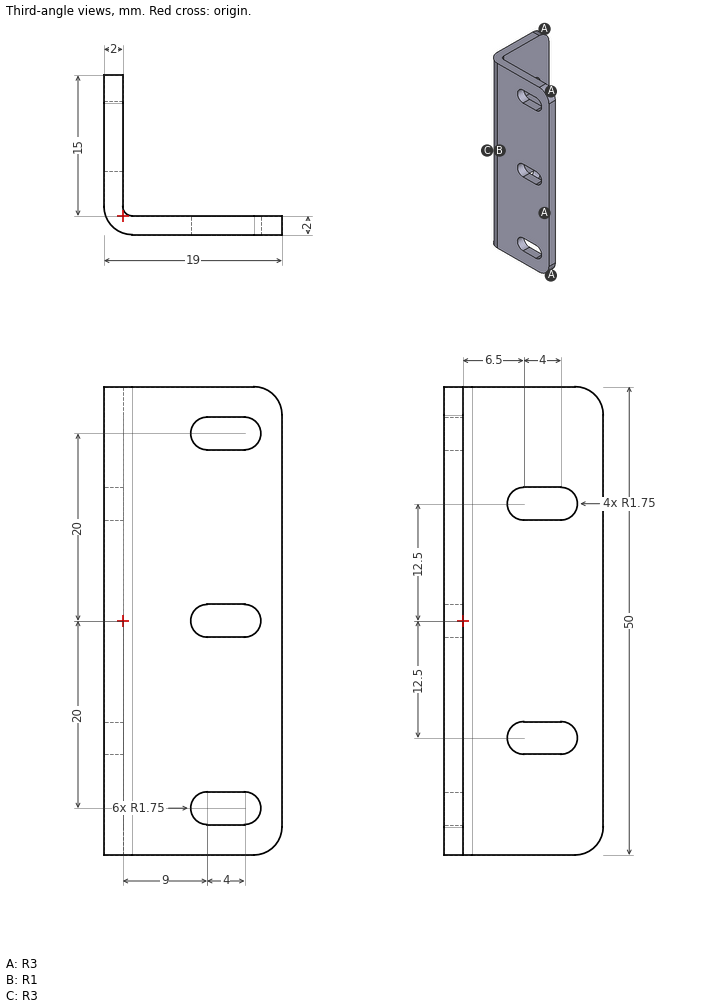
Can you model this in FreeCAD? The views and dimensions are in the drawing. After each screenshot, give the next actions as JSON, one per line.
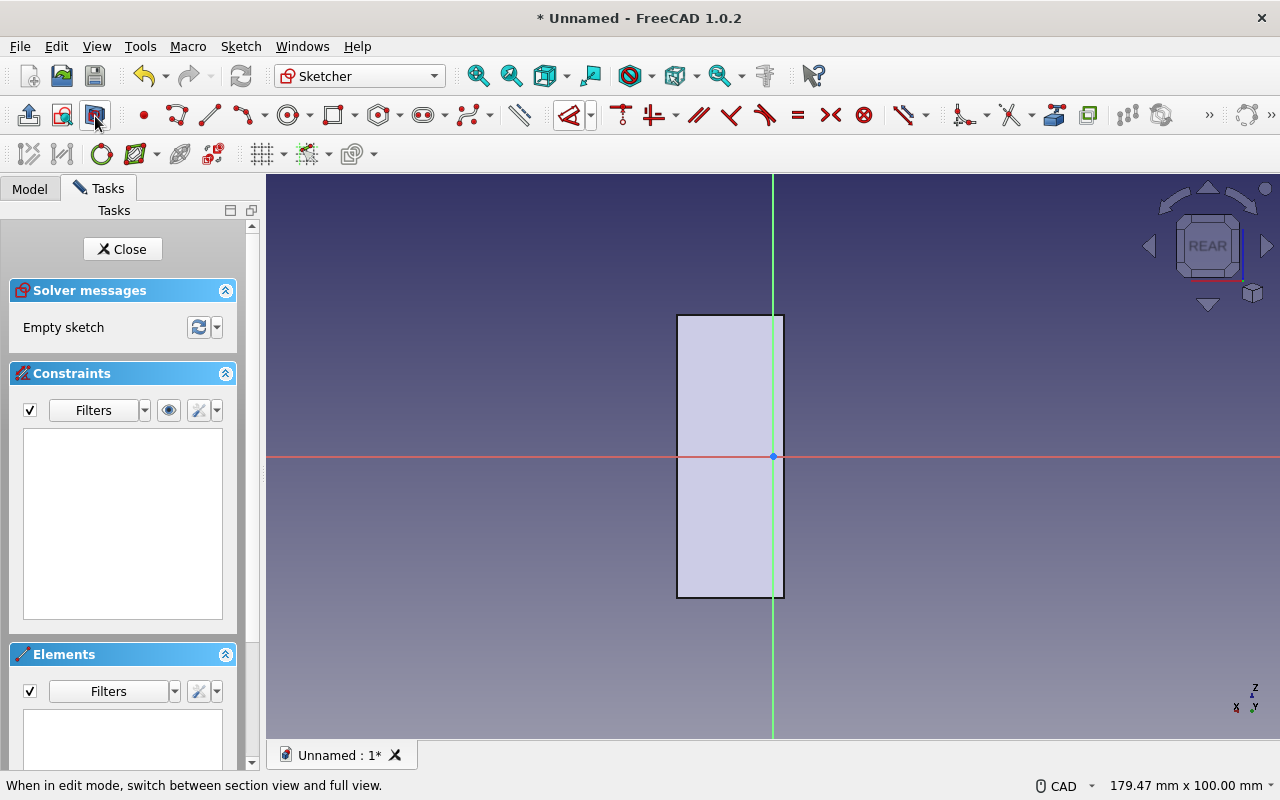
{"action": "scroll", "coordinate": [786, 456], "scroll_direction": "up", "scroll_amount": 2}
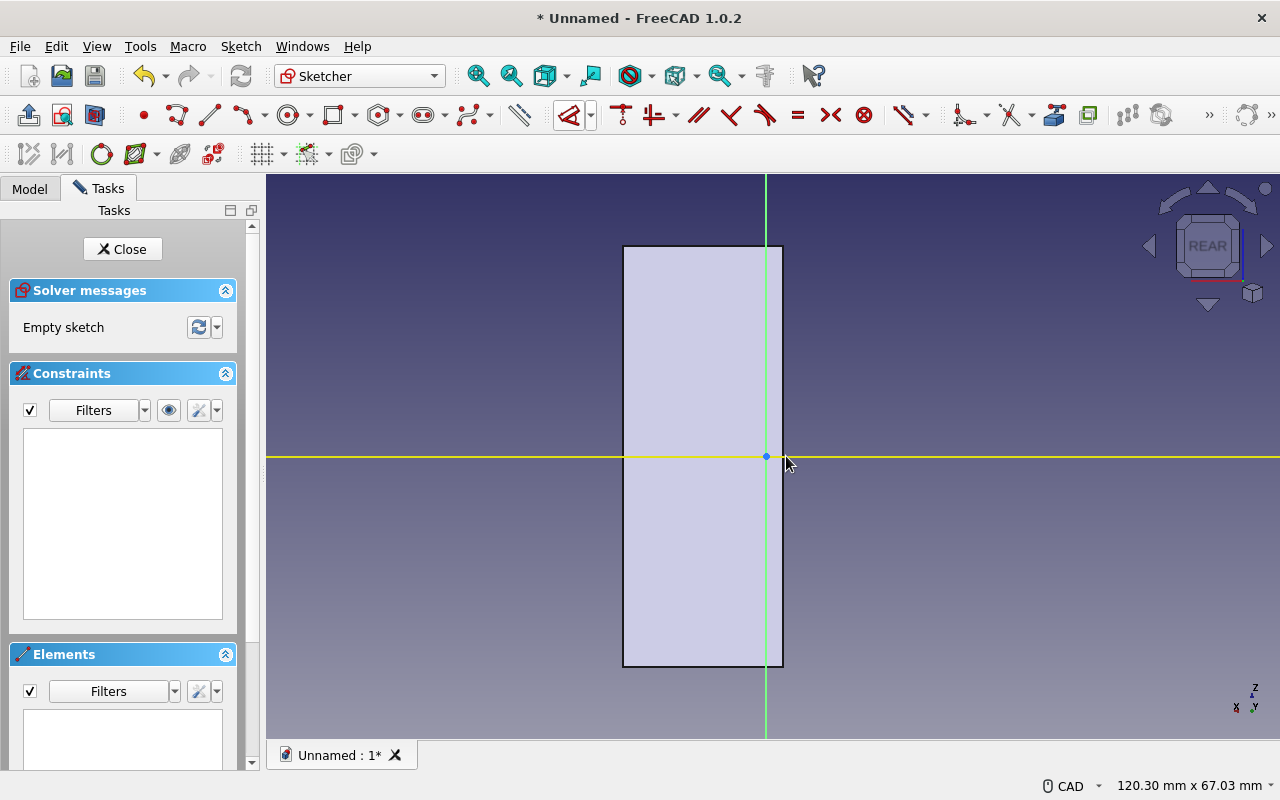
{"action": "key", "text": "g s"}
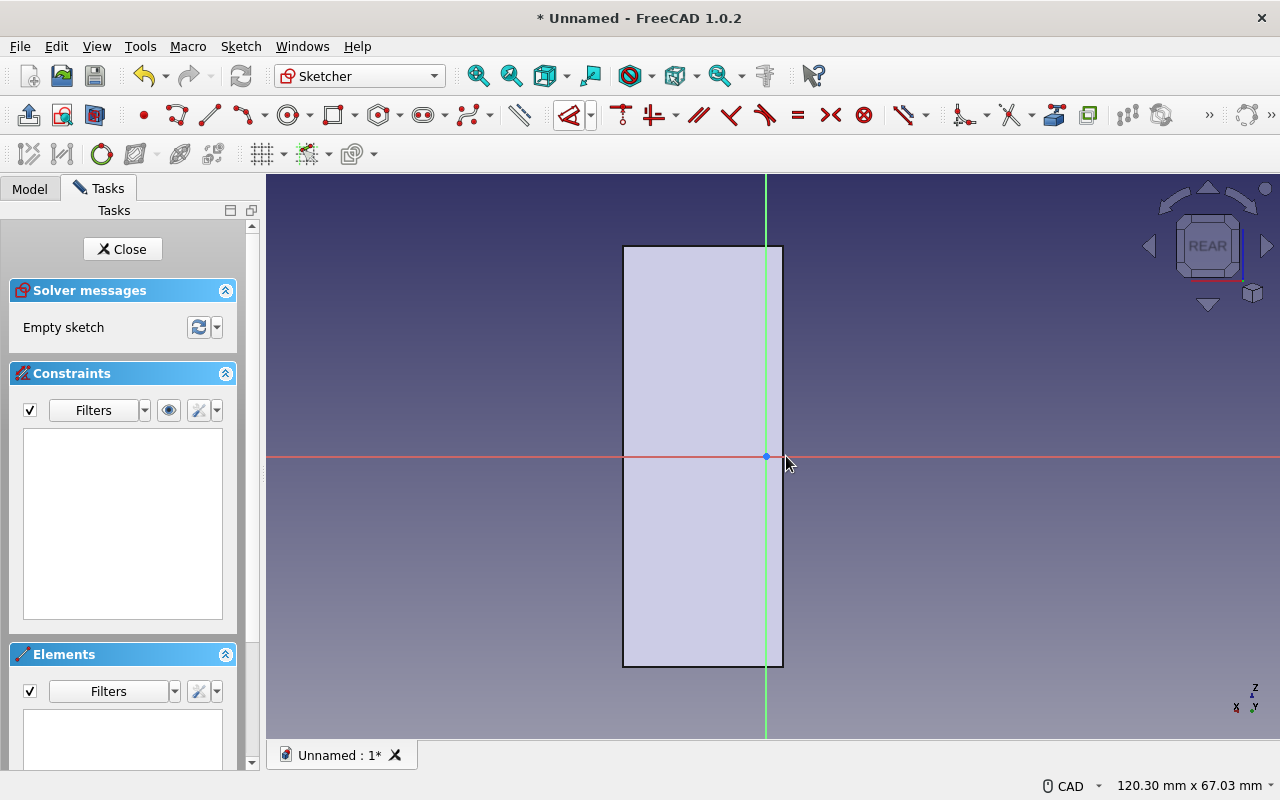
{"action": "scroll", "coordinate": [657, 625], "scroll_direction": "up", "scroll_amount": 3}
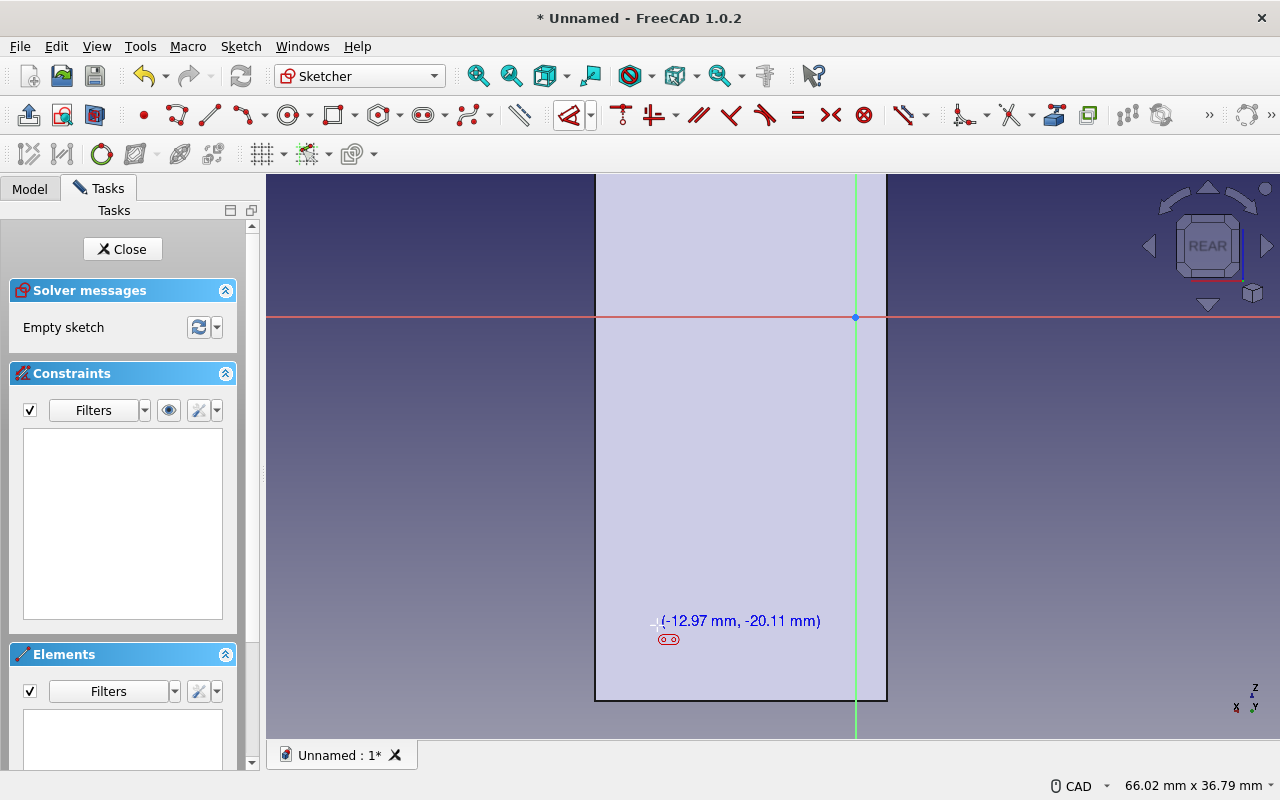
{"action": "left_click", "coordinate": [656, 624]}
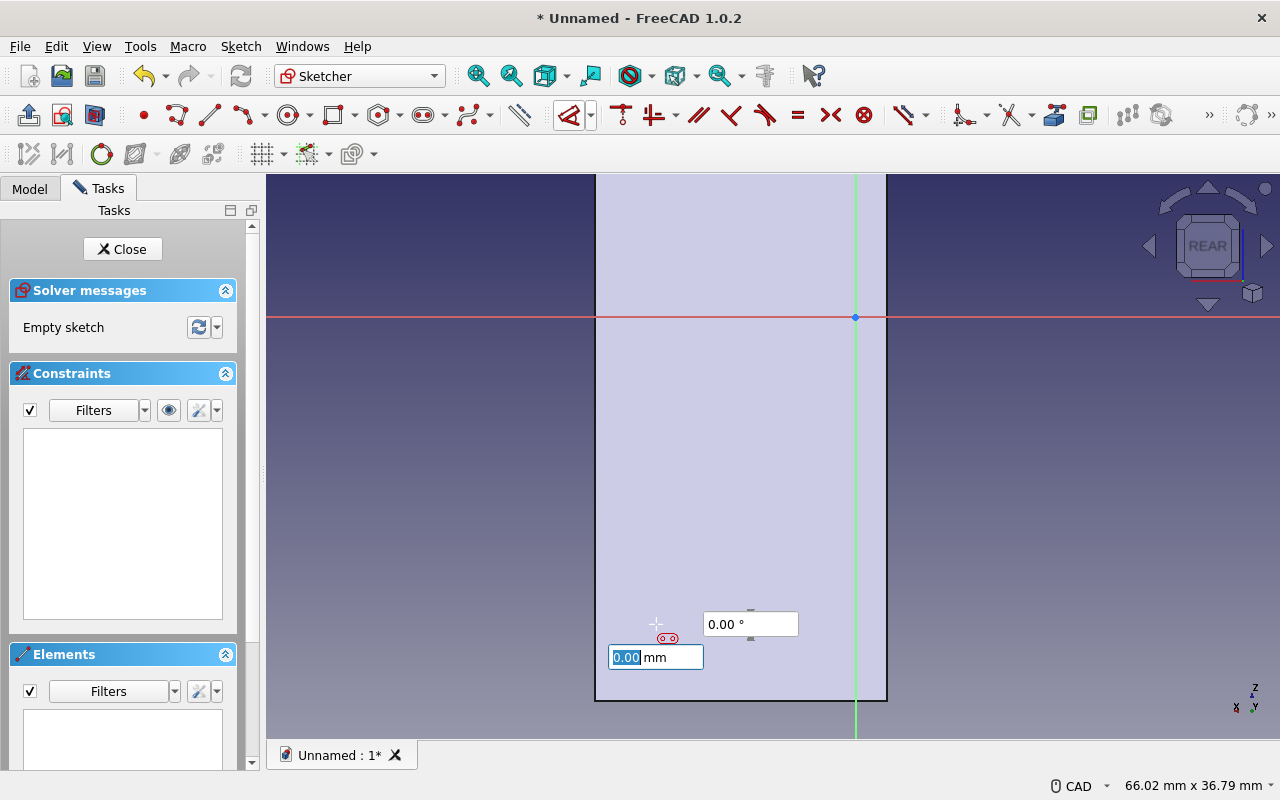
{"action": "left_click", "coordinate": [718, 624]}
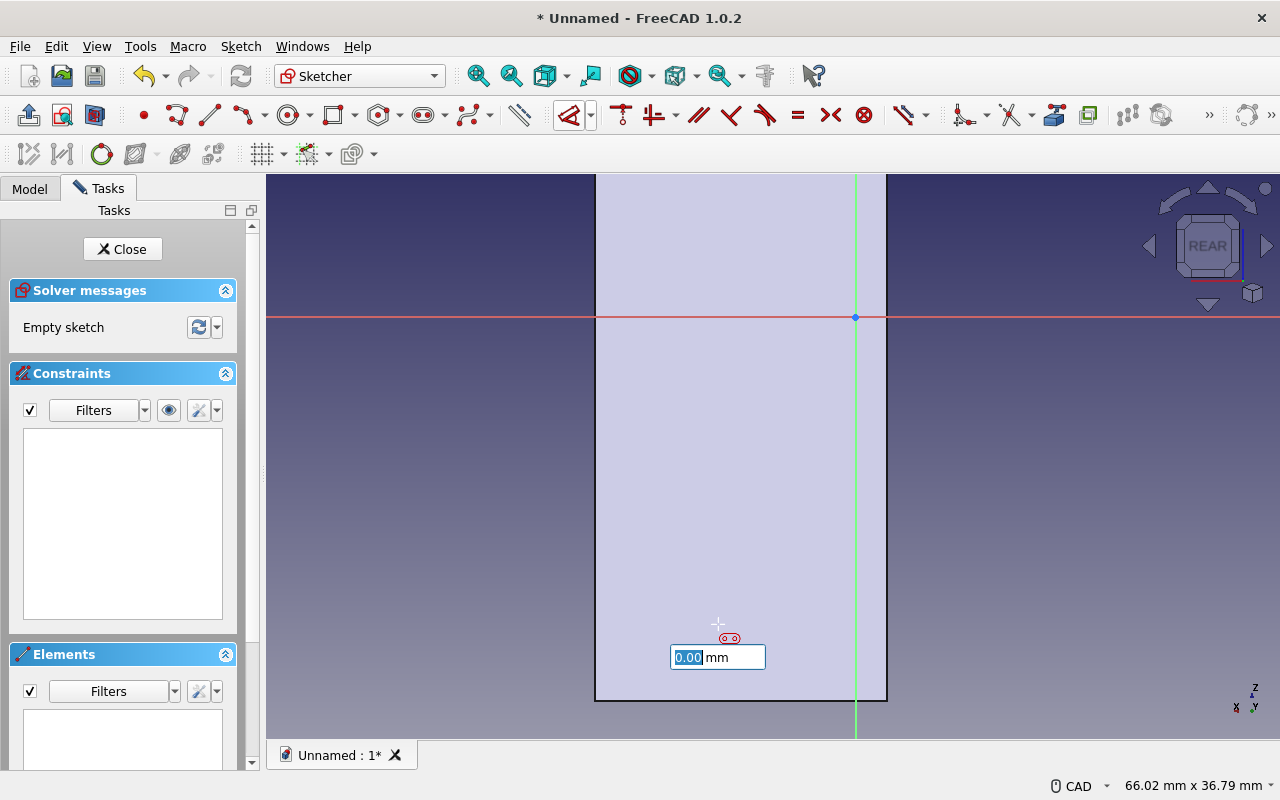
{"action": "left_click", "coordinate": [687, 651]}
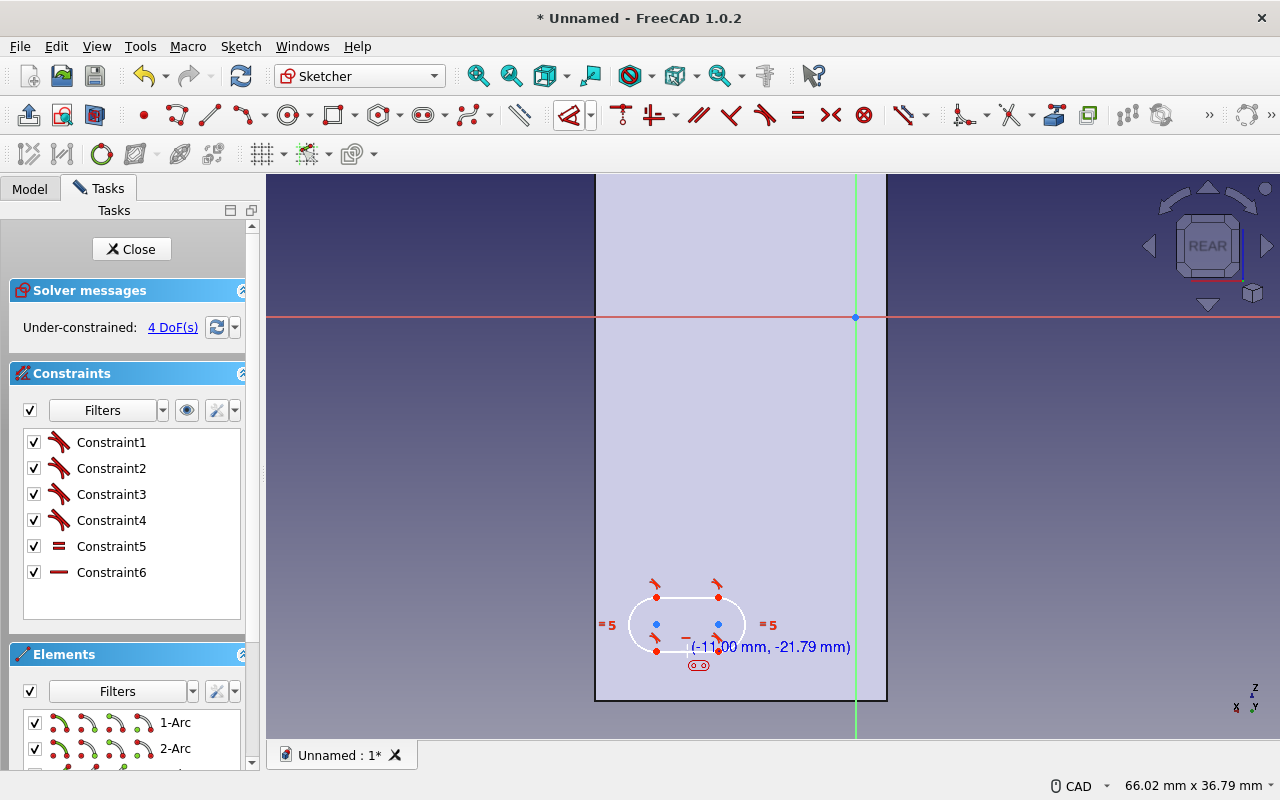
{"action": "scroll", "coordinate": [658, 626], "scroll_direction": "down", "scroll_amount": 3}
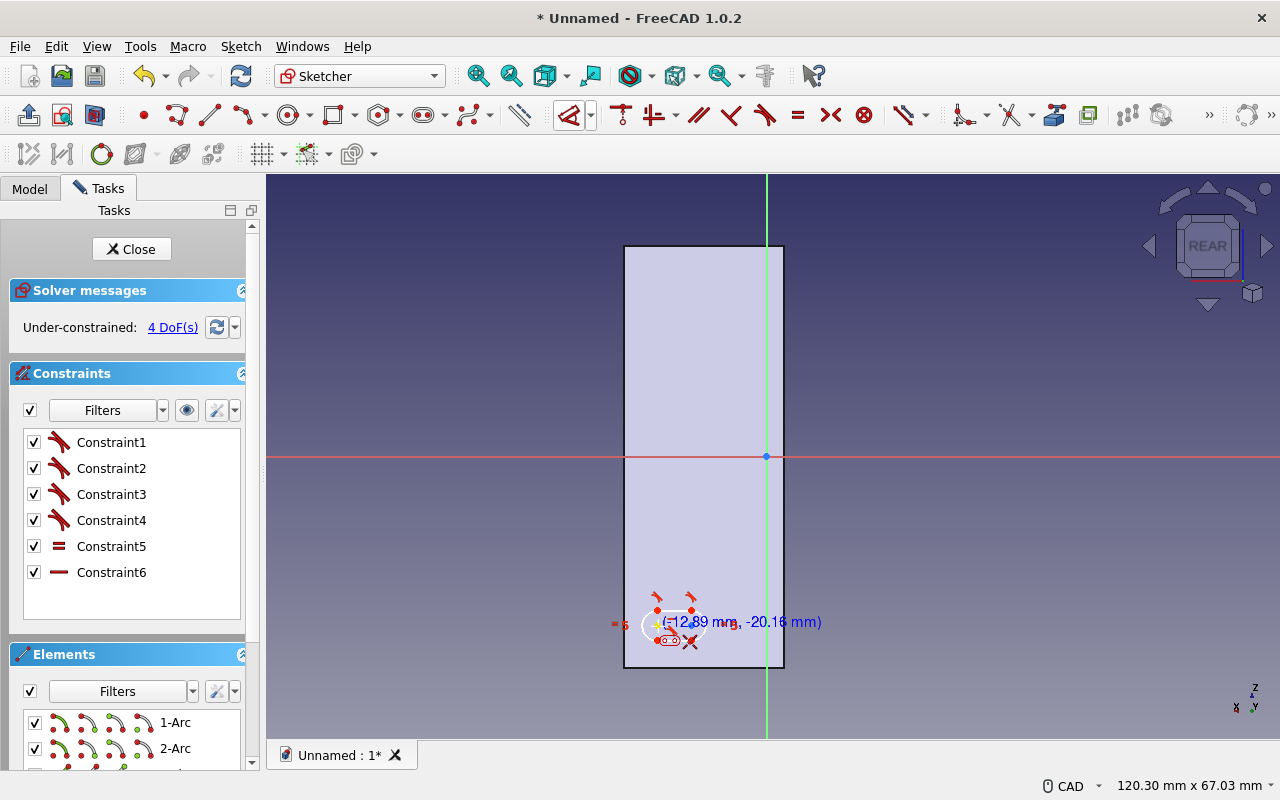
{"action": "scroll", "coordinate": [657, 288], "scroll_direction": "up", "scroll_amount": 3}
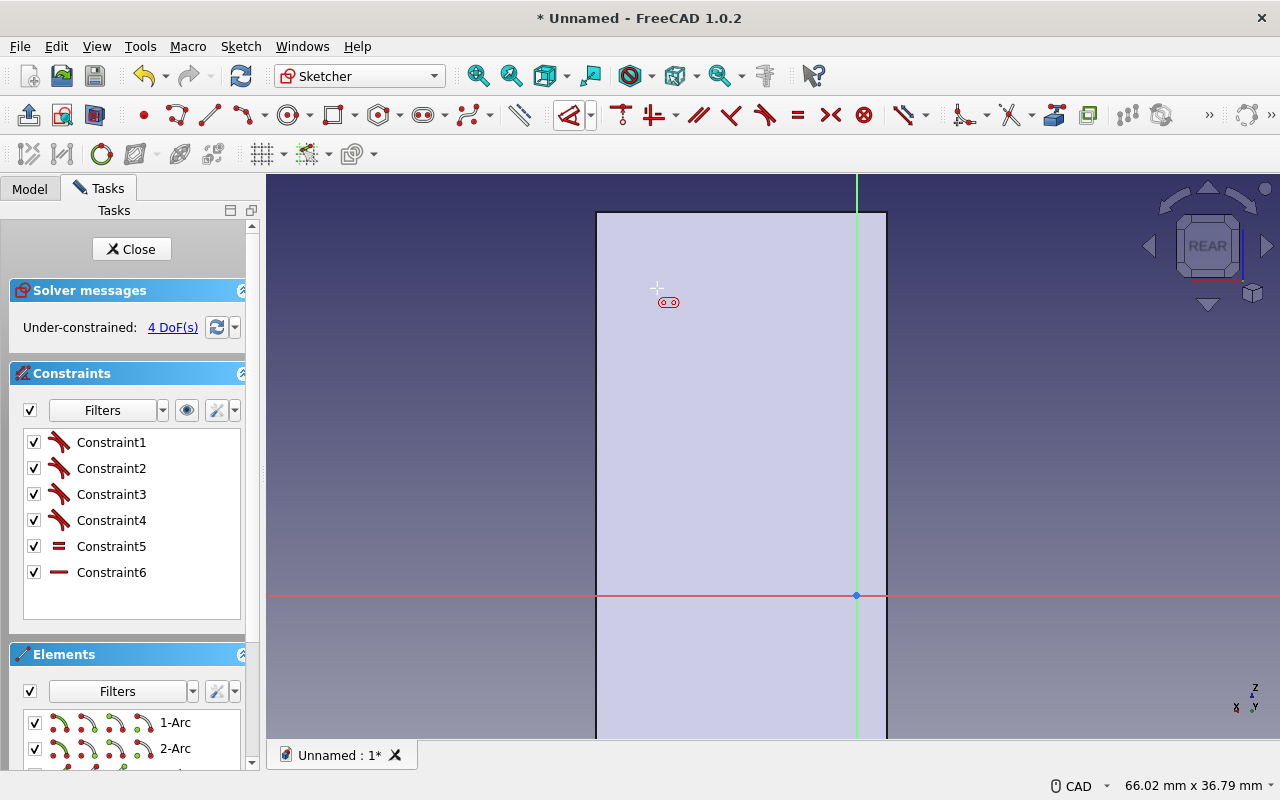
{"action": "left_click", "coordinate": [657, 289]}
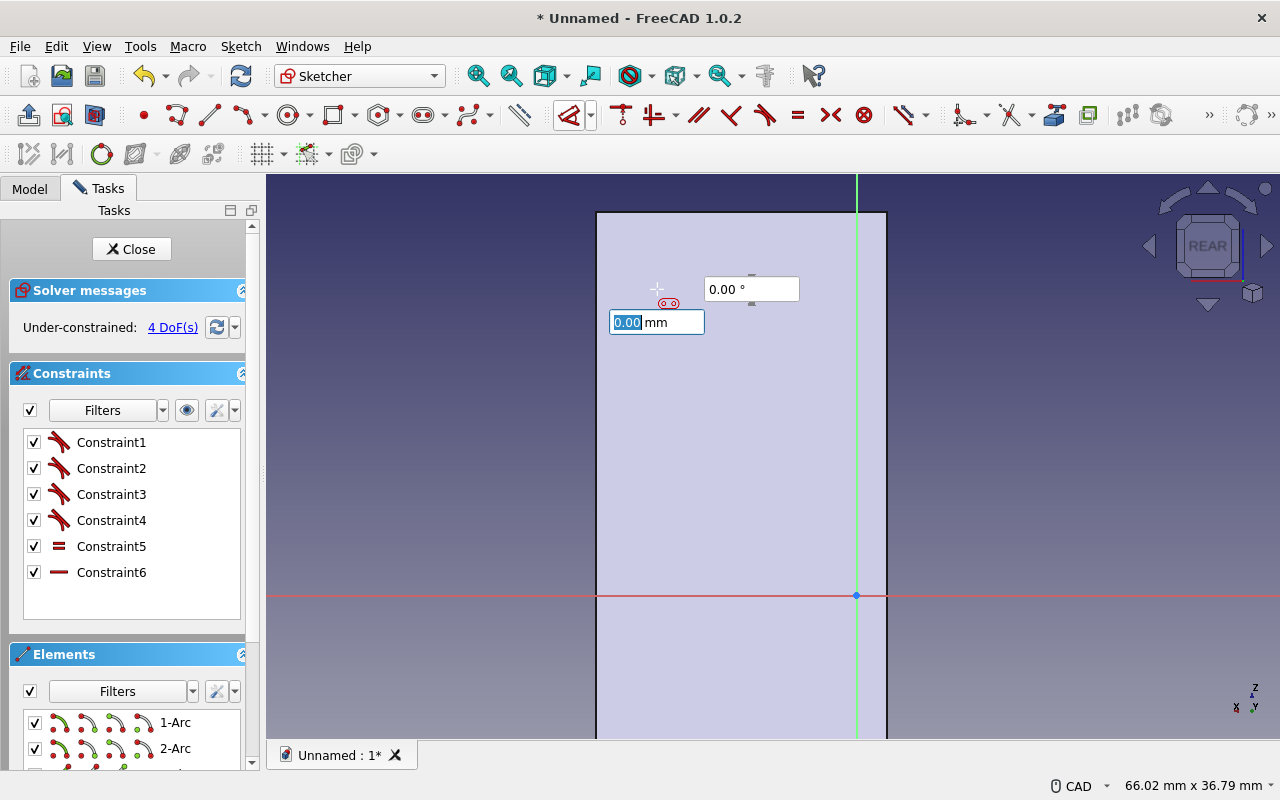
{"action": "left_click", "coordinate": [719, 289]}